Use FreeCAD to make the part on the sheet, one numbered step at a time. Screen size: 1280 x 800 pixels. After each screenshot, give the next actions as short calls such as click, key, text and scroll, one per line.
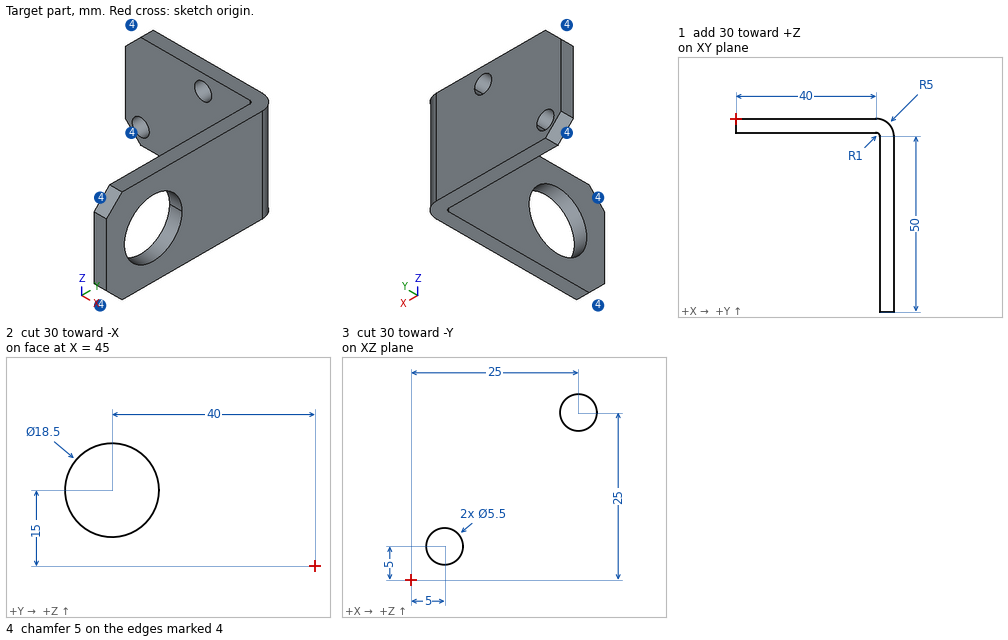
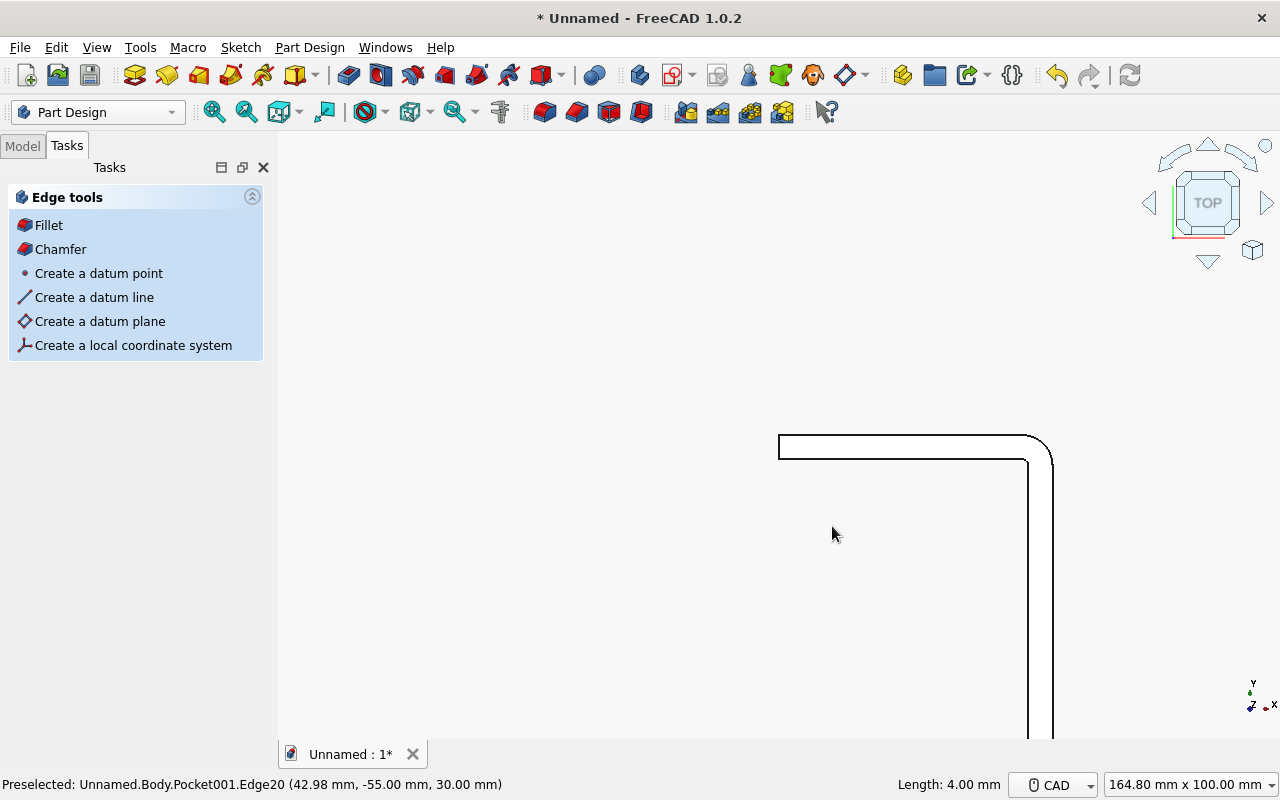
key(v)
key(f)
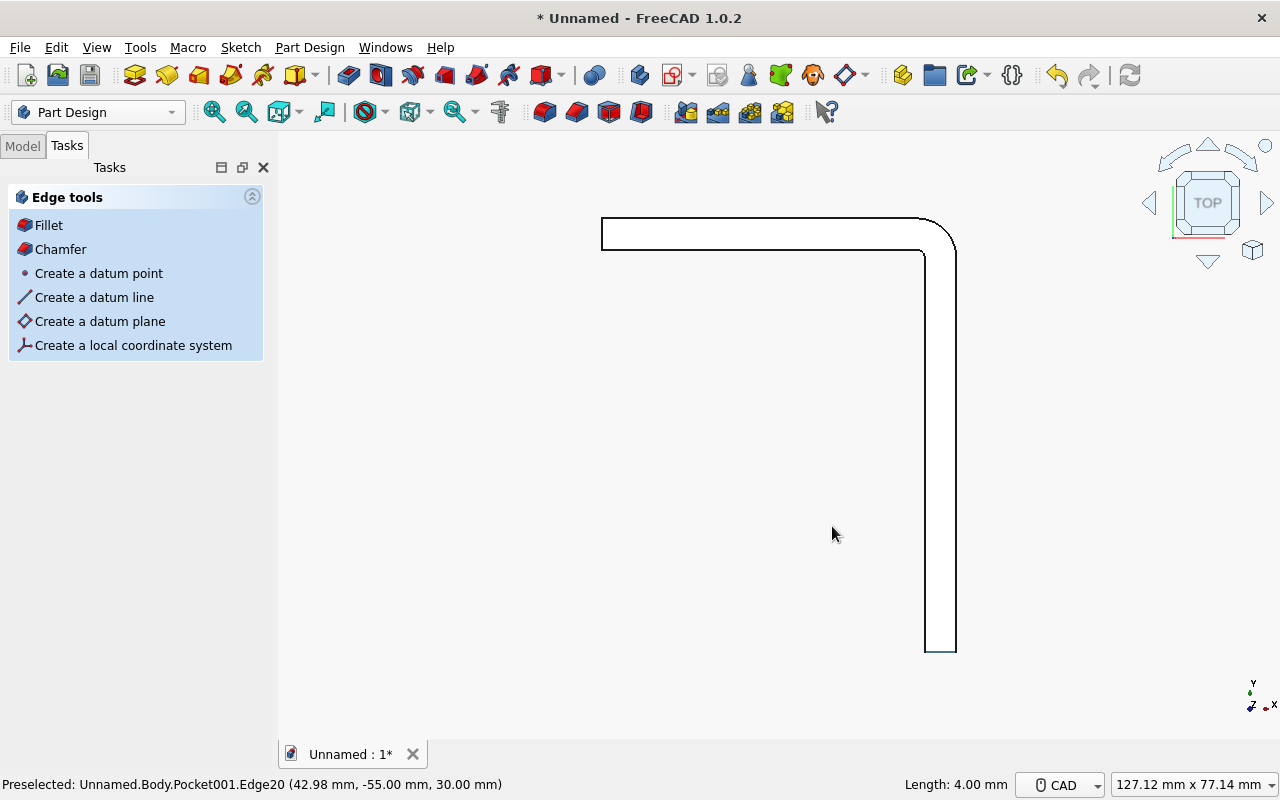
click(602, 233, ctrl)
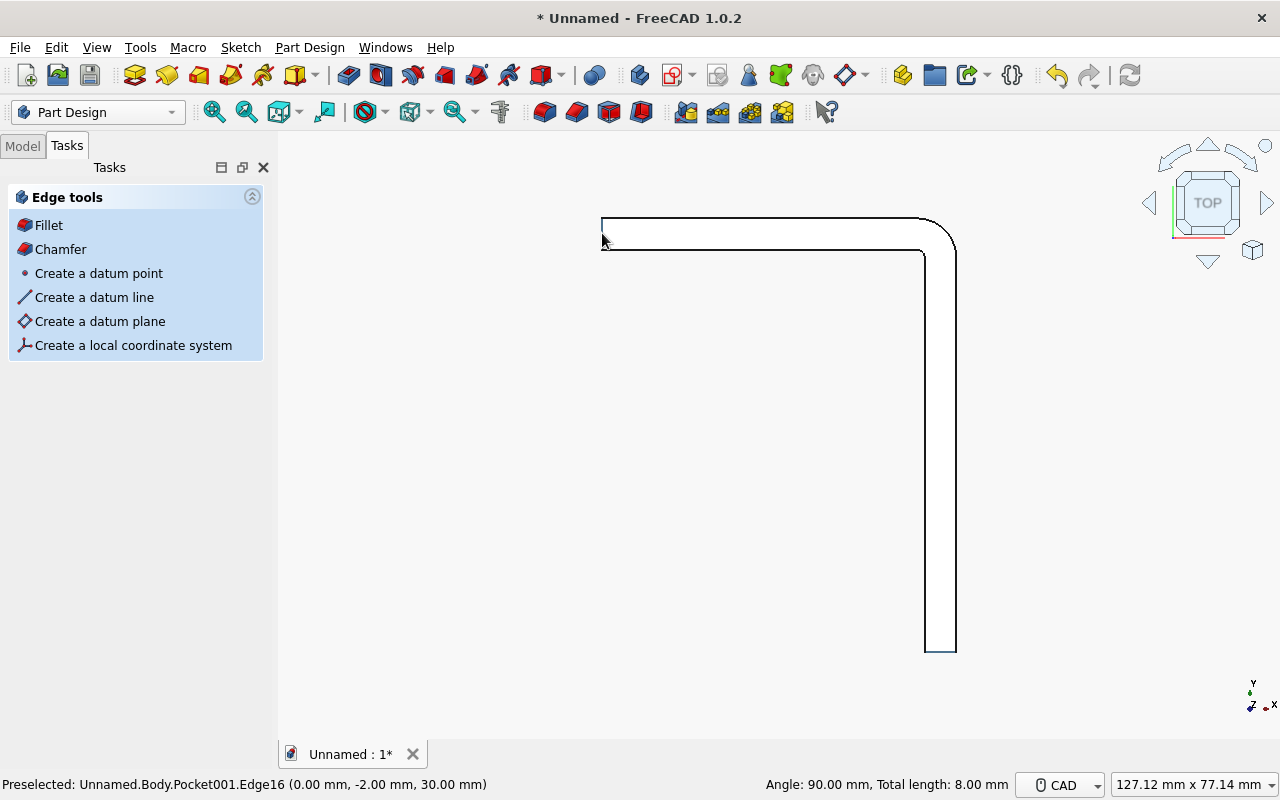
key(1)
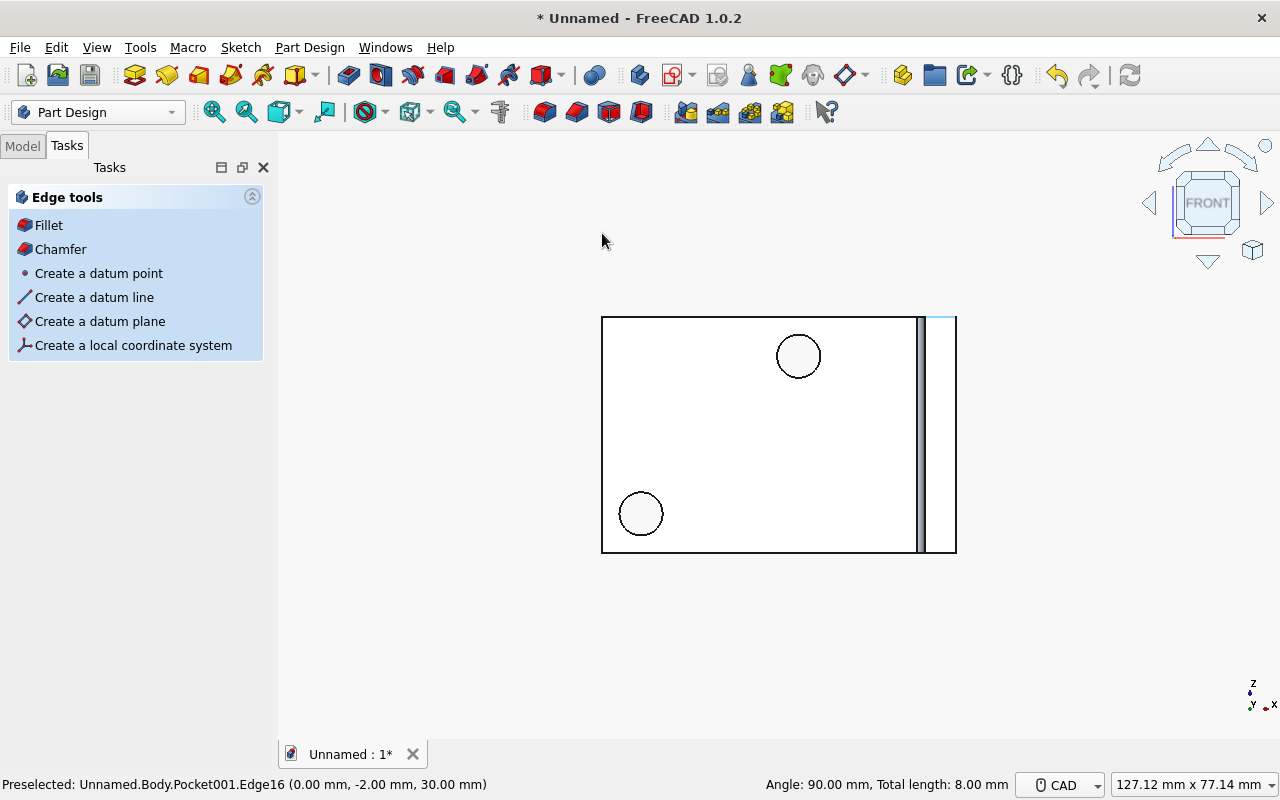
click(216, 112)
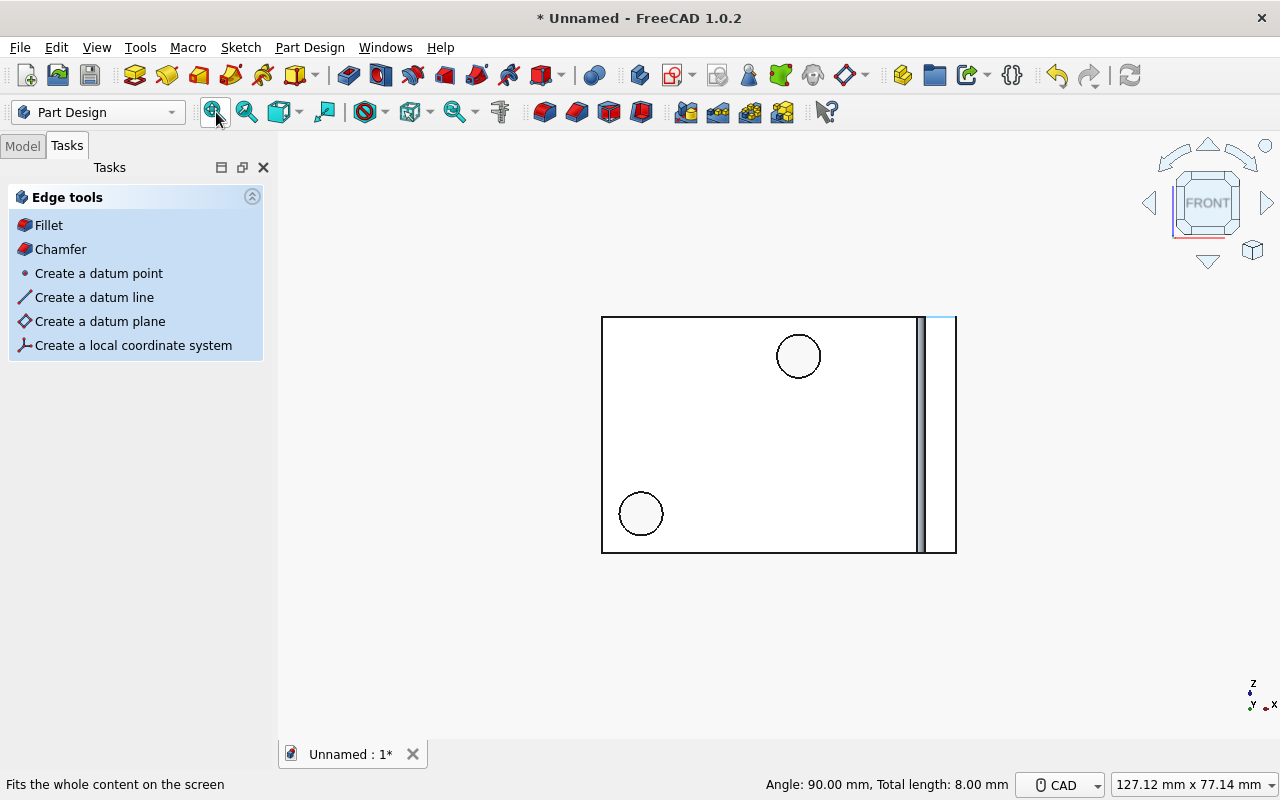
click(941, 552, ctrl)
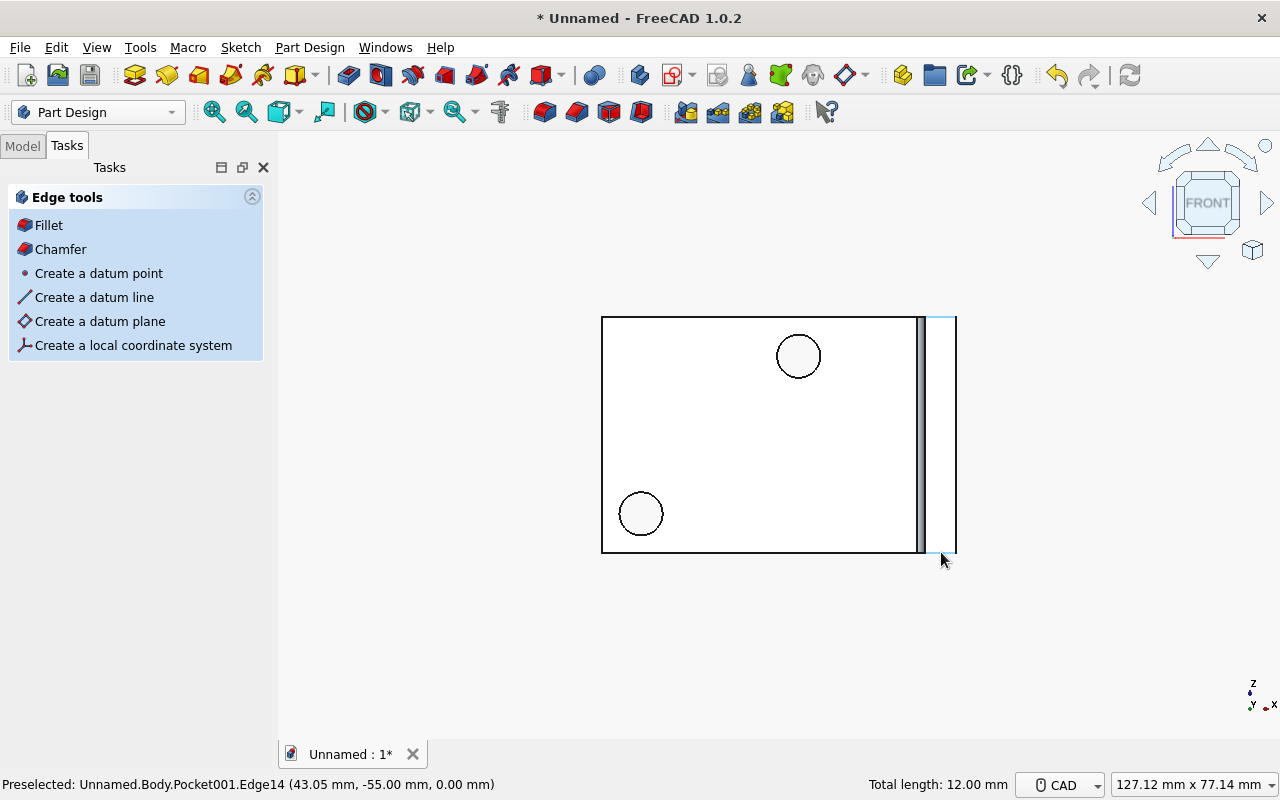
key(3)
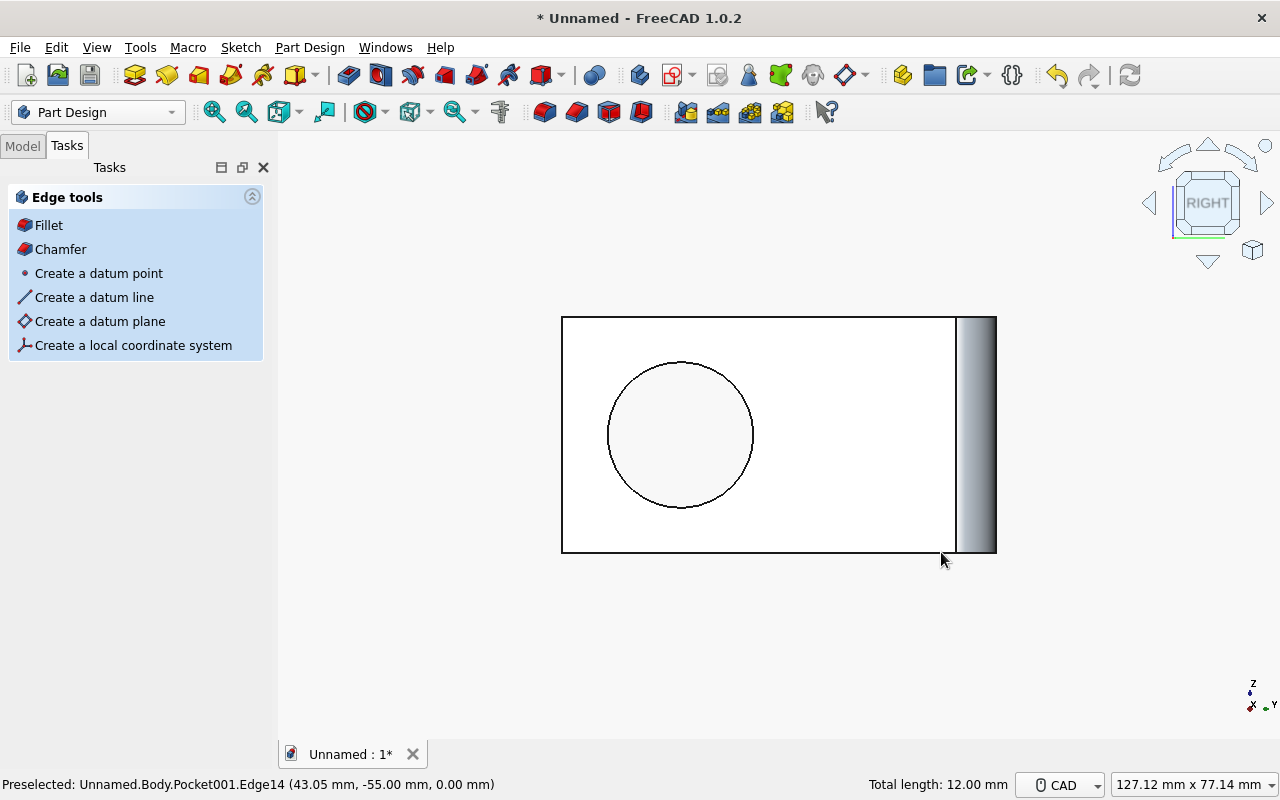
key(v)
key(f)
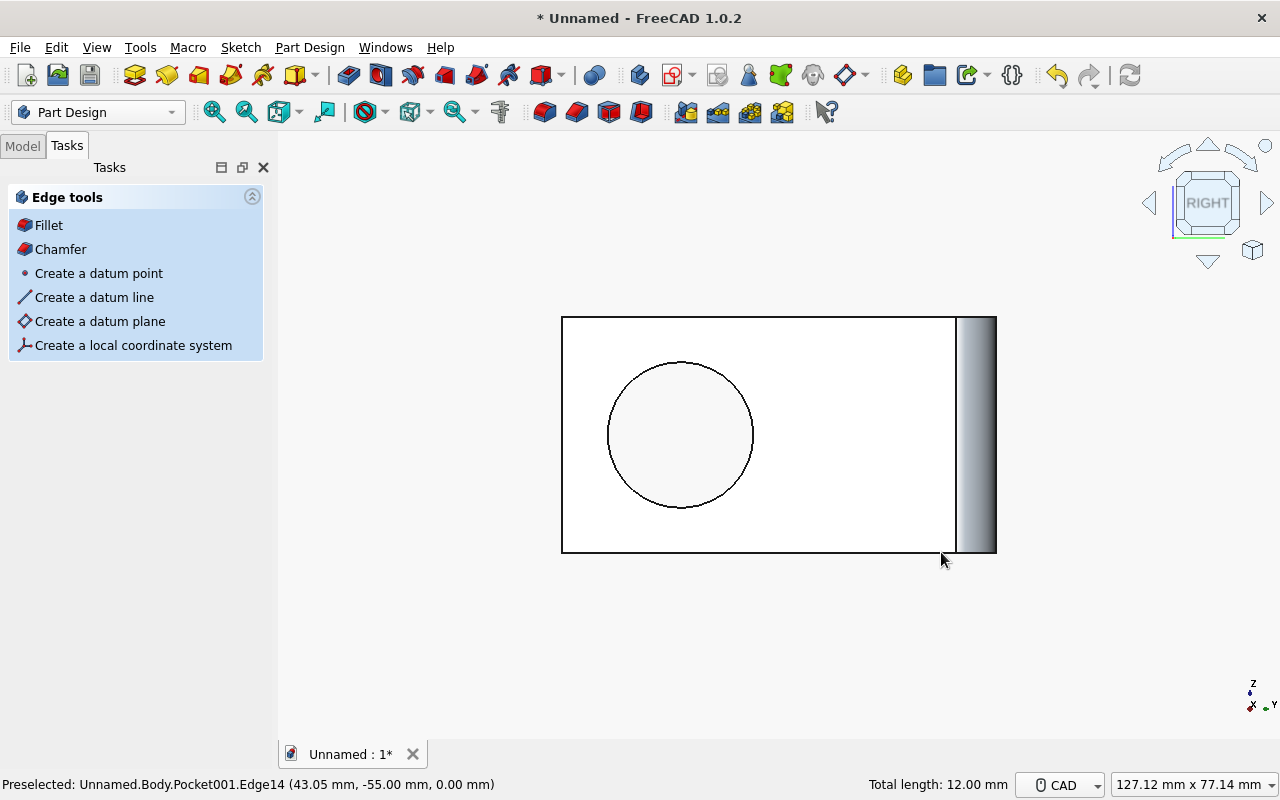
key(5)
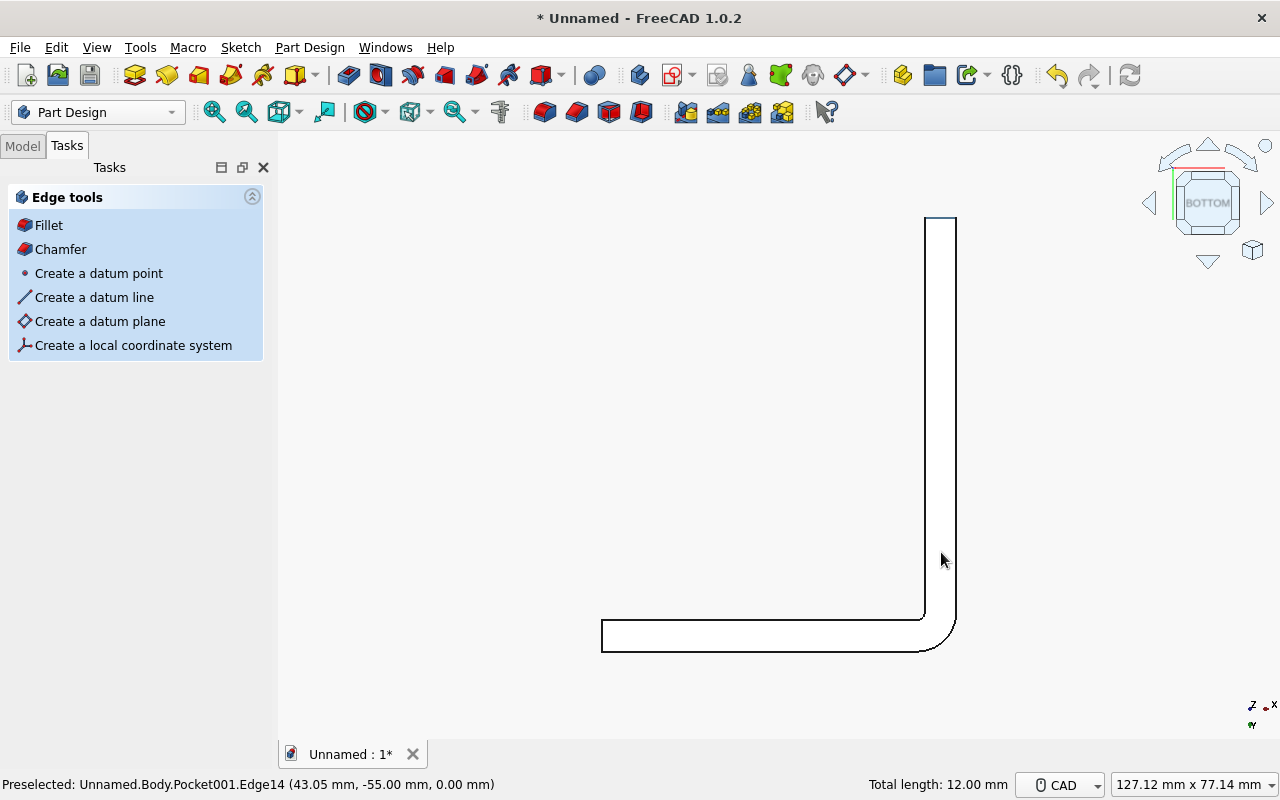
click(602, 635, ctrl)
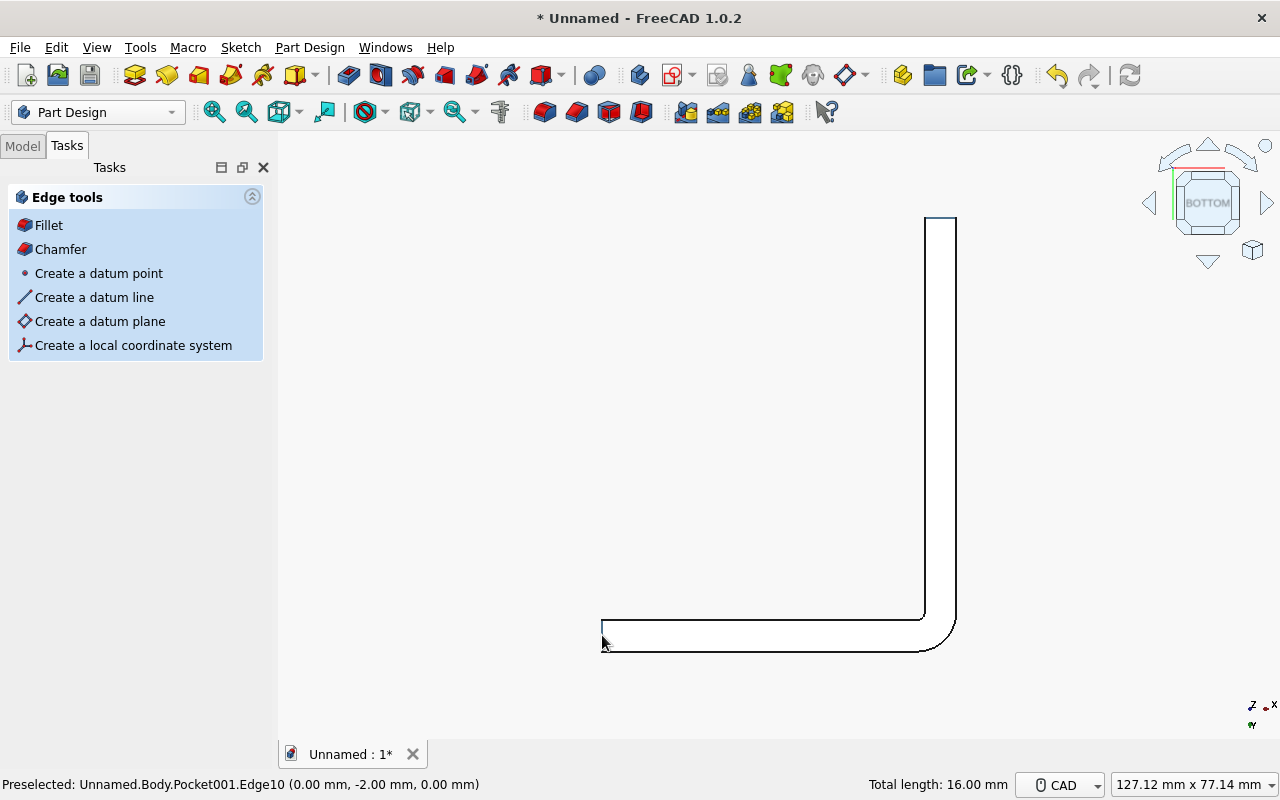
click(578, 112)